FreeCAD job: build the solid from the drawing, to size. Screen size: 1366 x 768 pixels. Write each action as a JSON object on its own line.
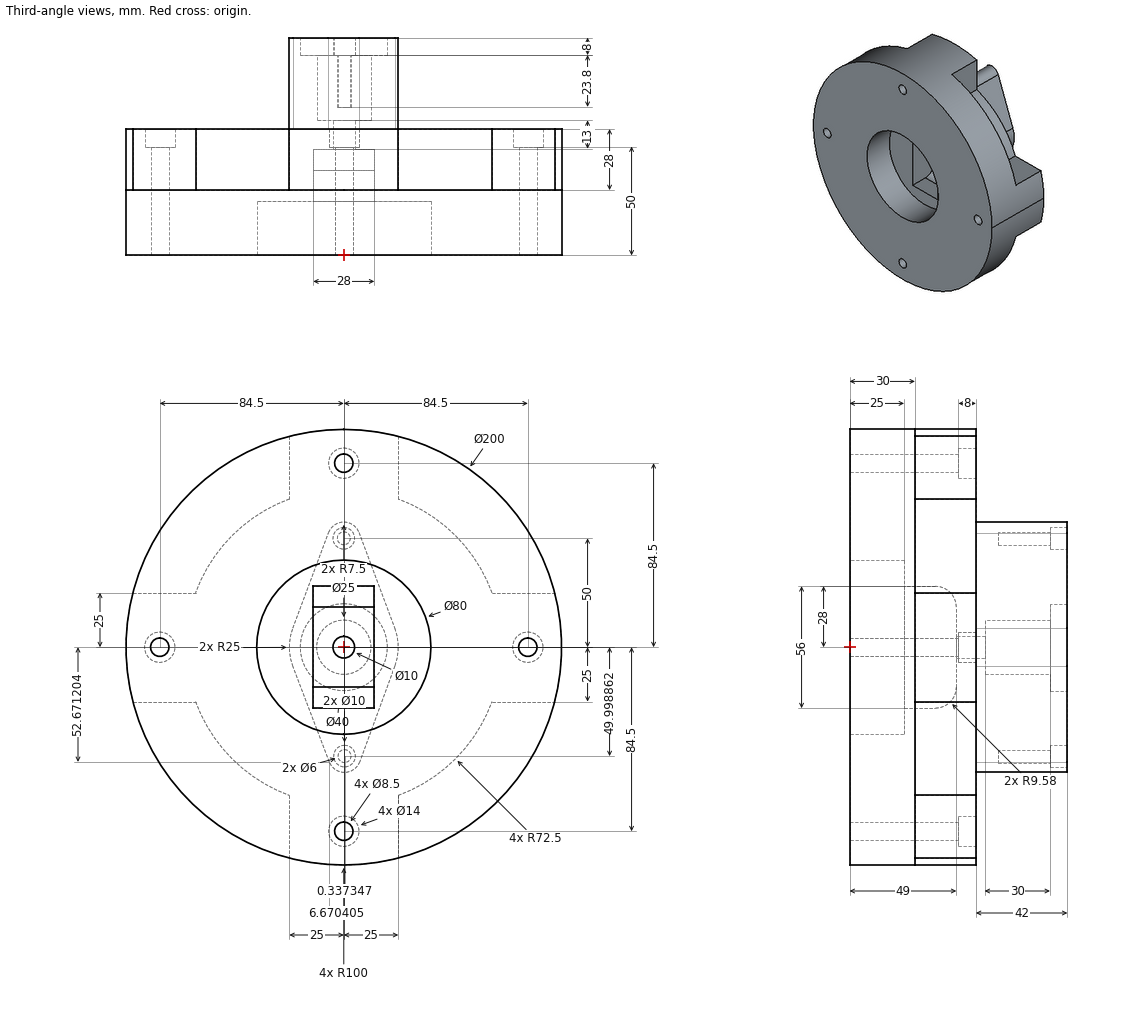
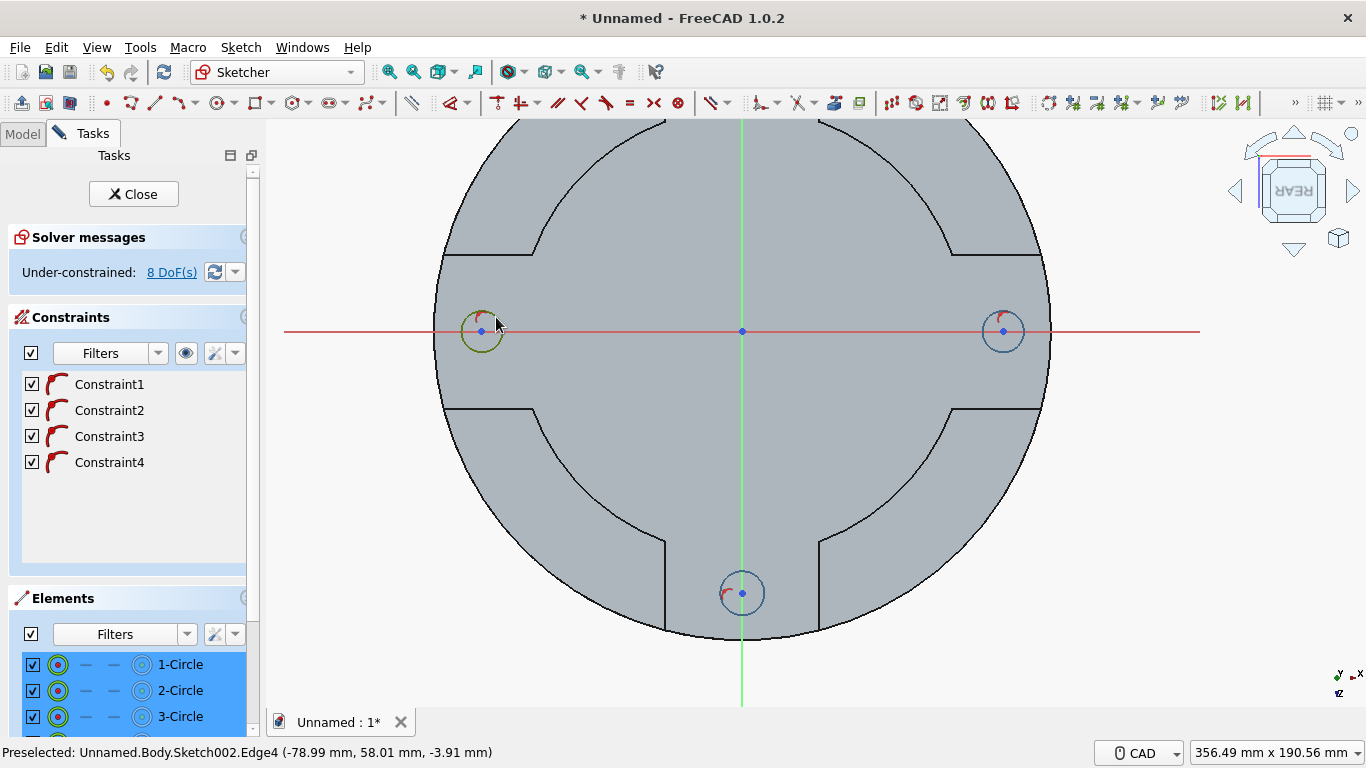
{"action": "key", "text": "e"}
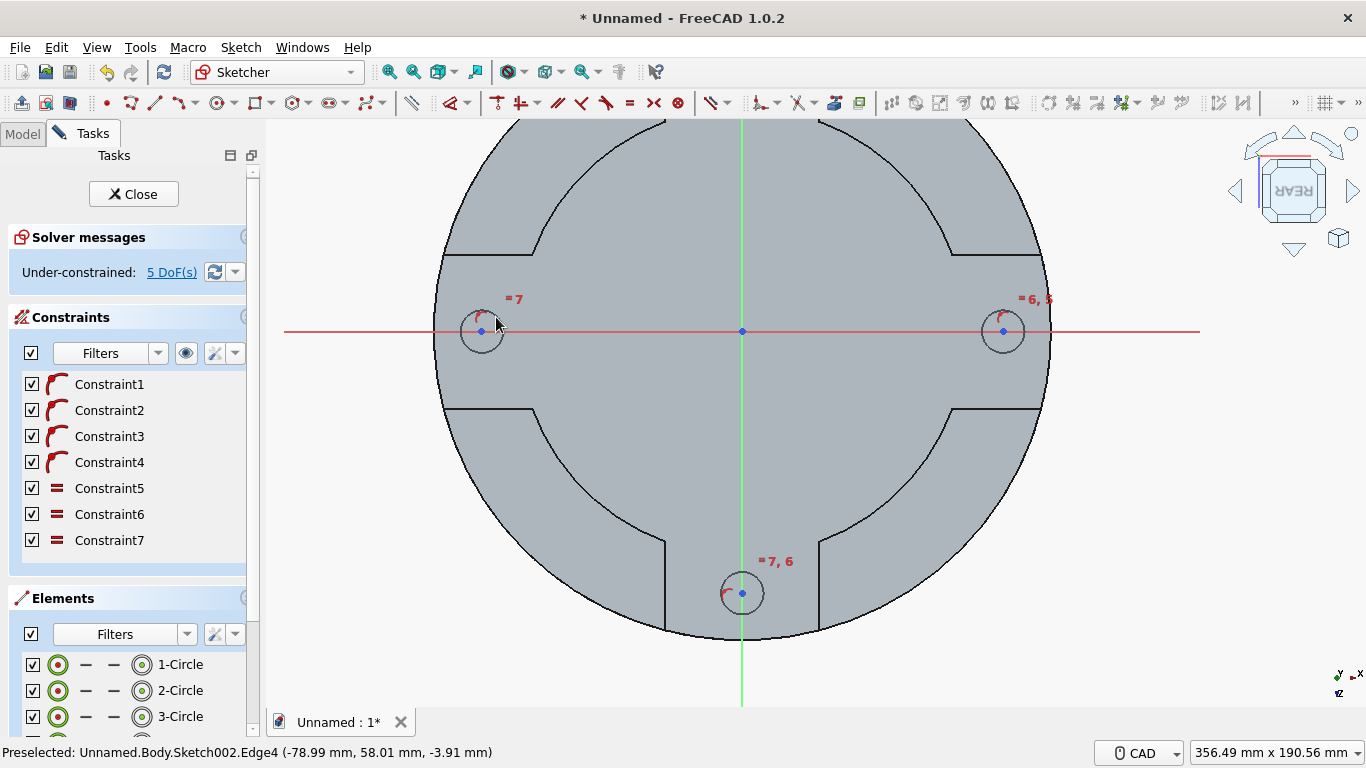
{"action": "left_click", "coordinate": [450, 104]}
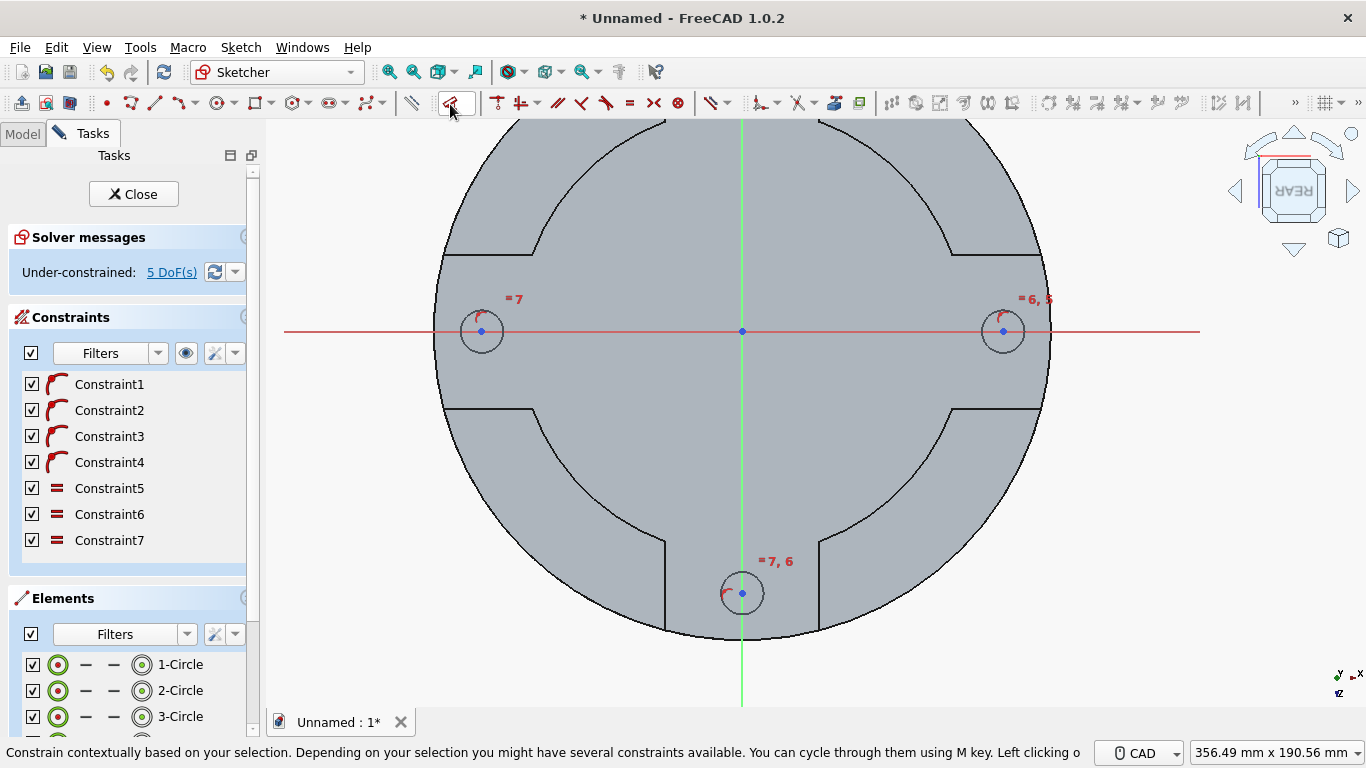
{"action": "scroll", "coordinate": [758, 578], "scroll_direction": "down", "scroll_amount": 2}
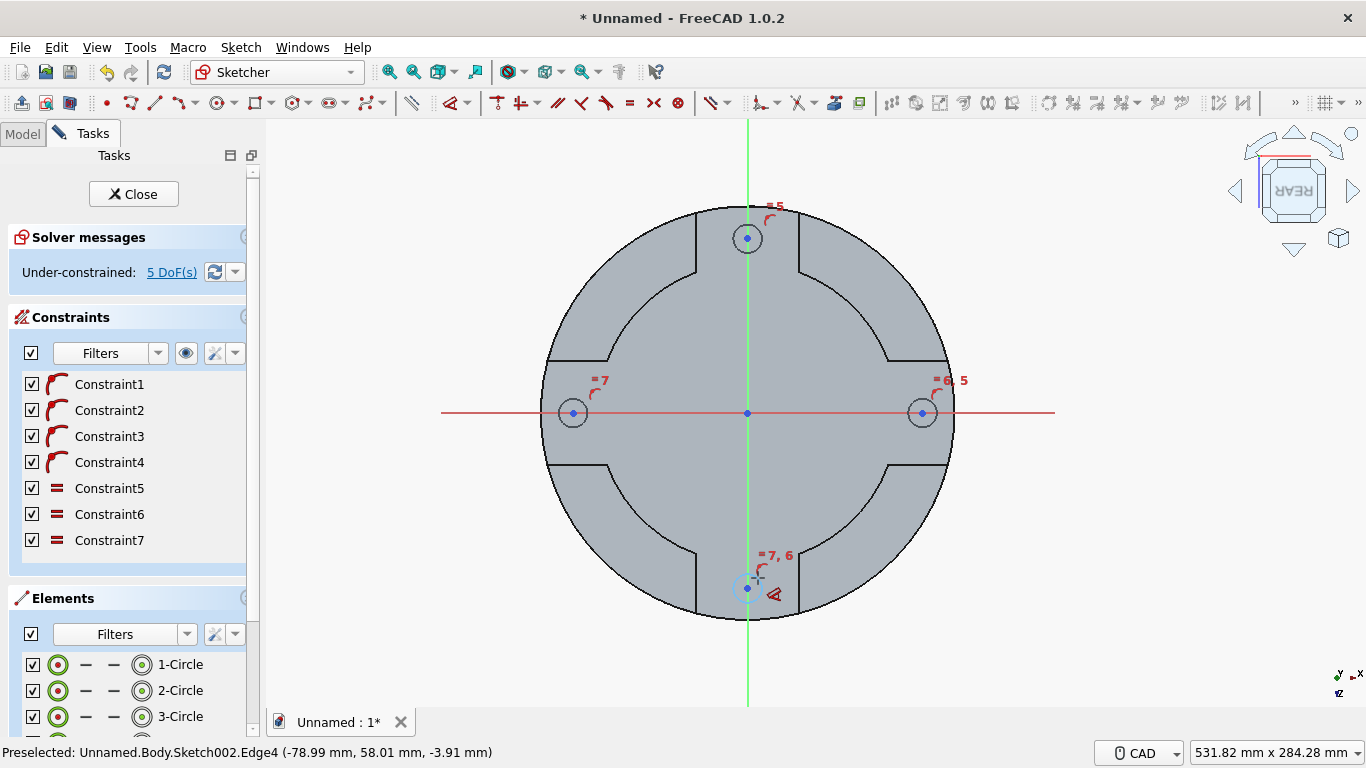
{"action": "scroll", "coordinate": [758, 229], "scroll_direction": "up", "scroll_amount": 2}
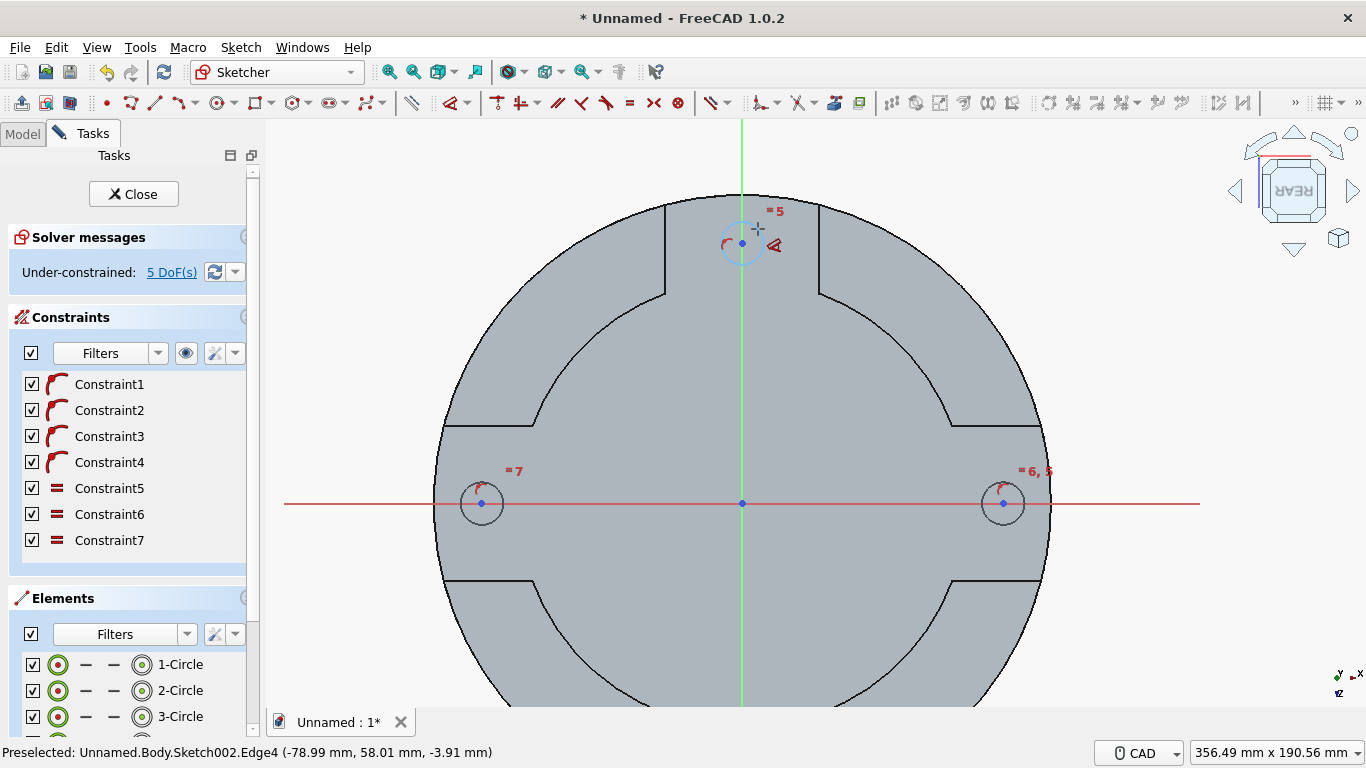
{"action": "left_click", "coordinate": [757, 228]}
{"action": "left_click", "coordinate": [779, 205]}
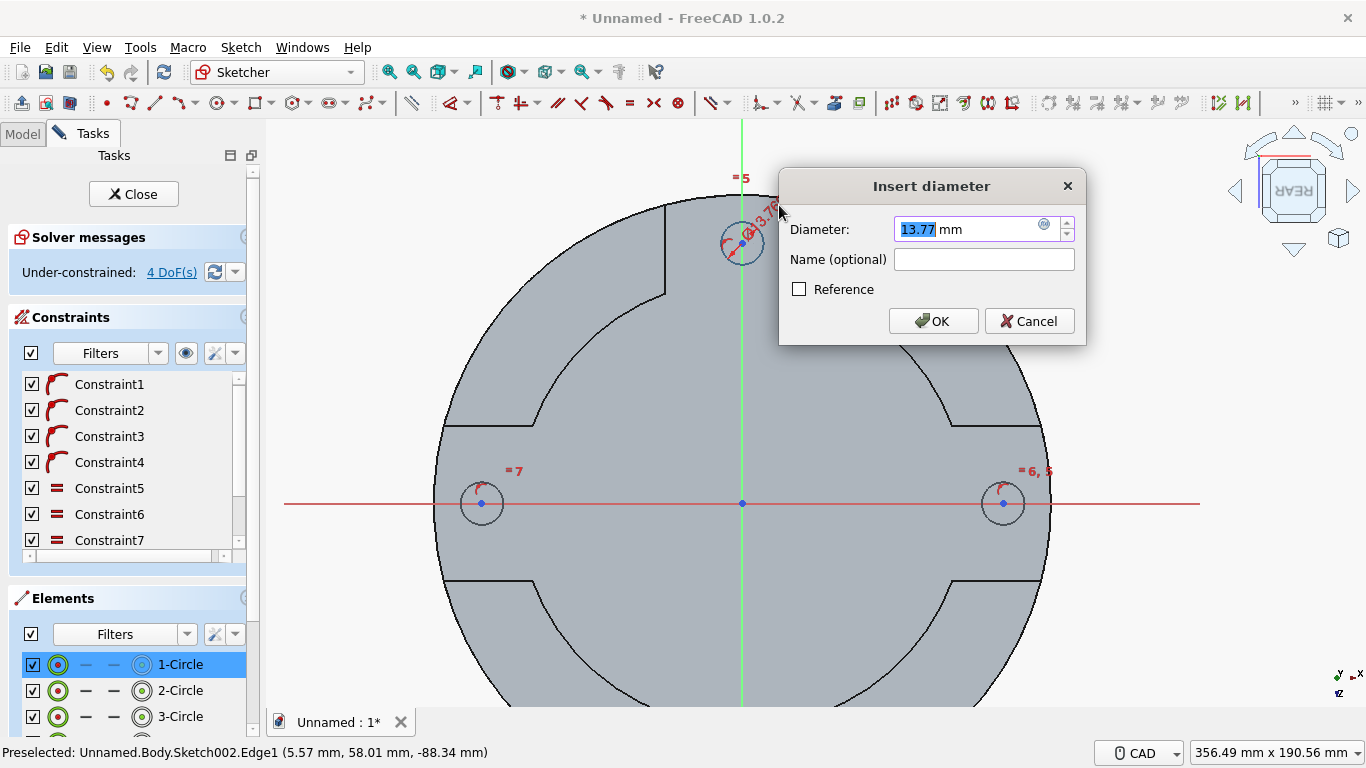
{"action": "type", "text": "14"}
{"action": "key", "text": "Return"}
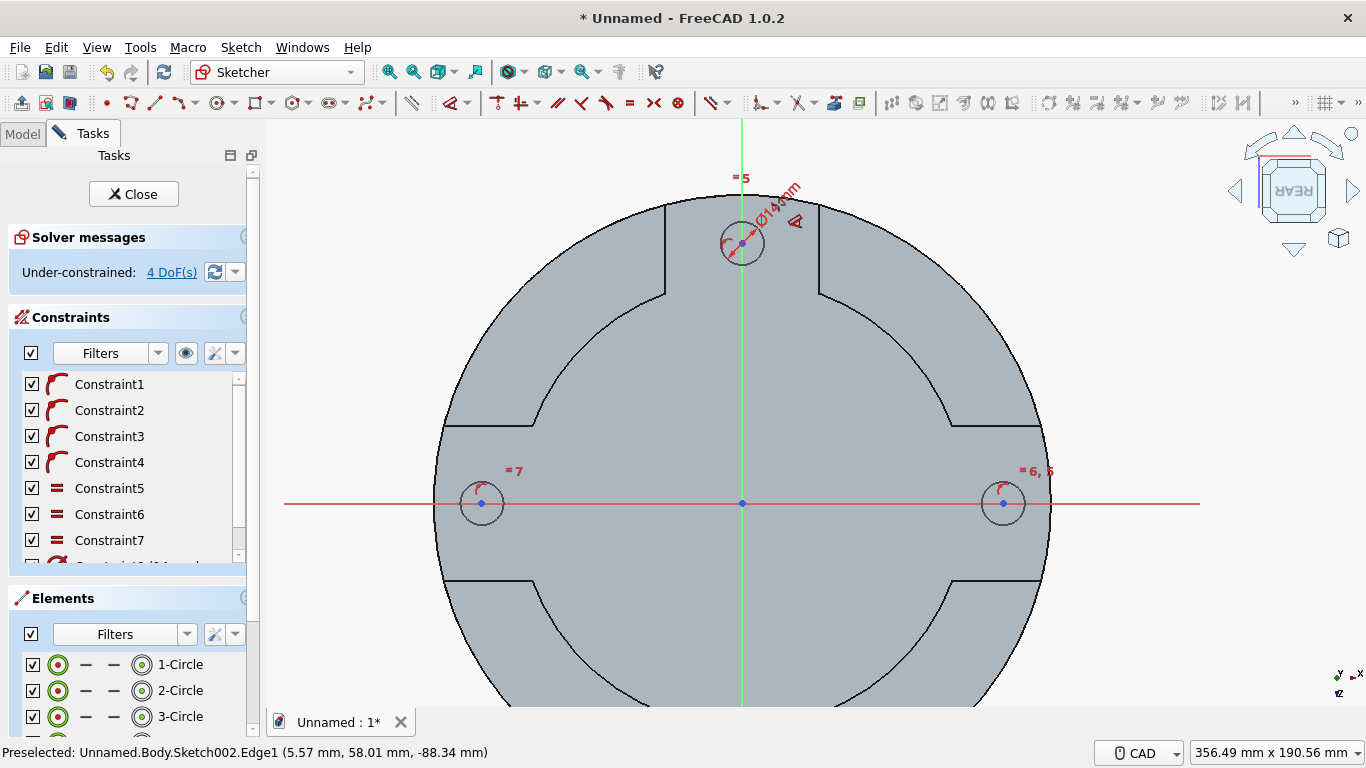
{"action": "left_click", "coordinate": [742, 243]}
{"action": "left_click", "coordinate": [776, 374]}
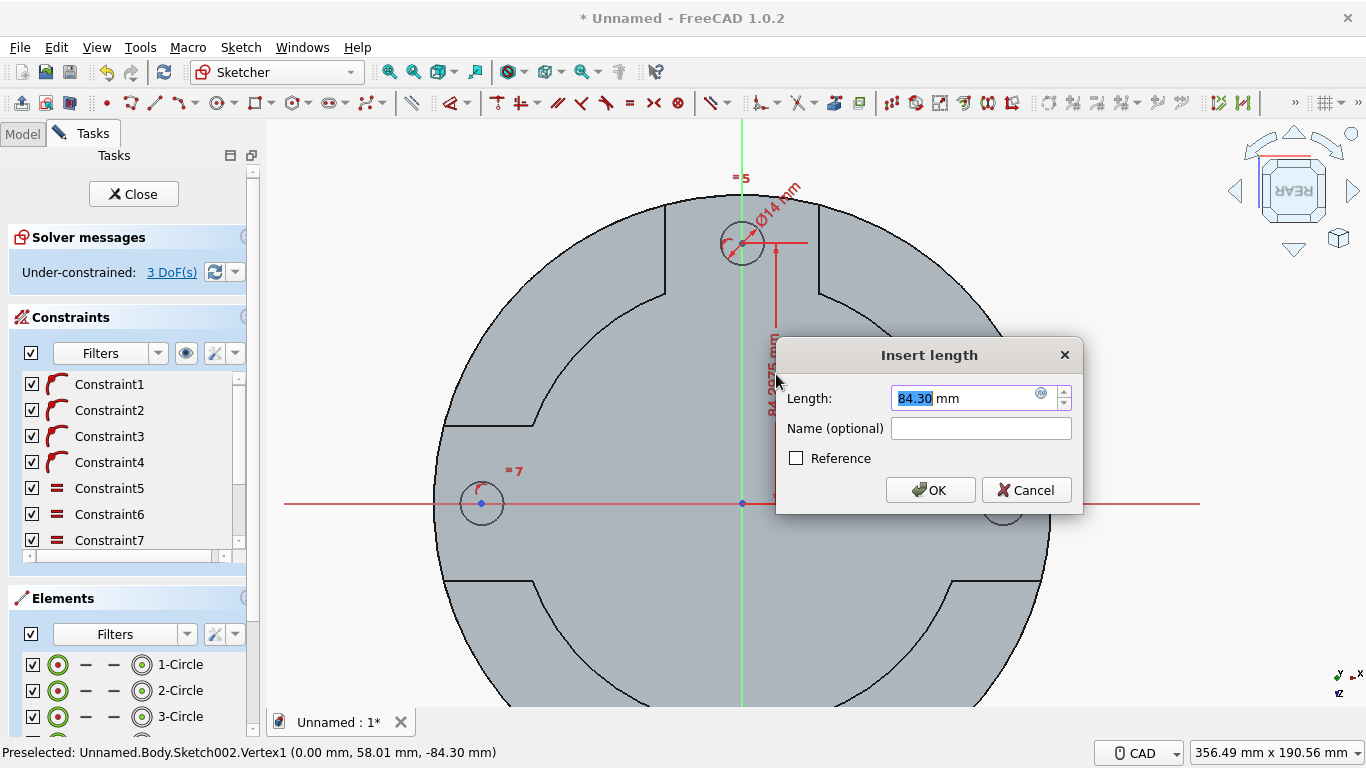
{"action": "type", "text": "84.5"}
{"action": "key", "text": "Return"}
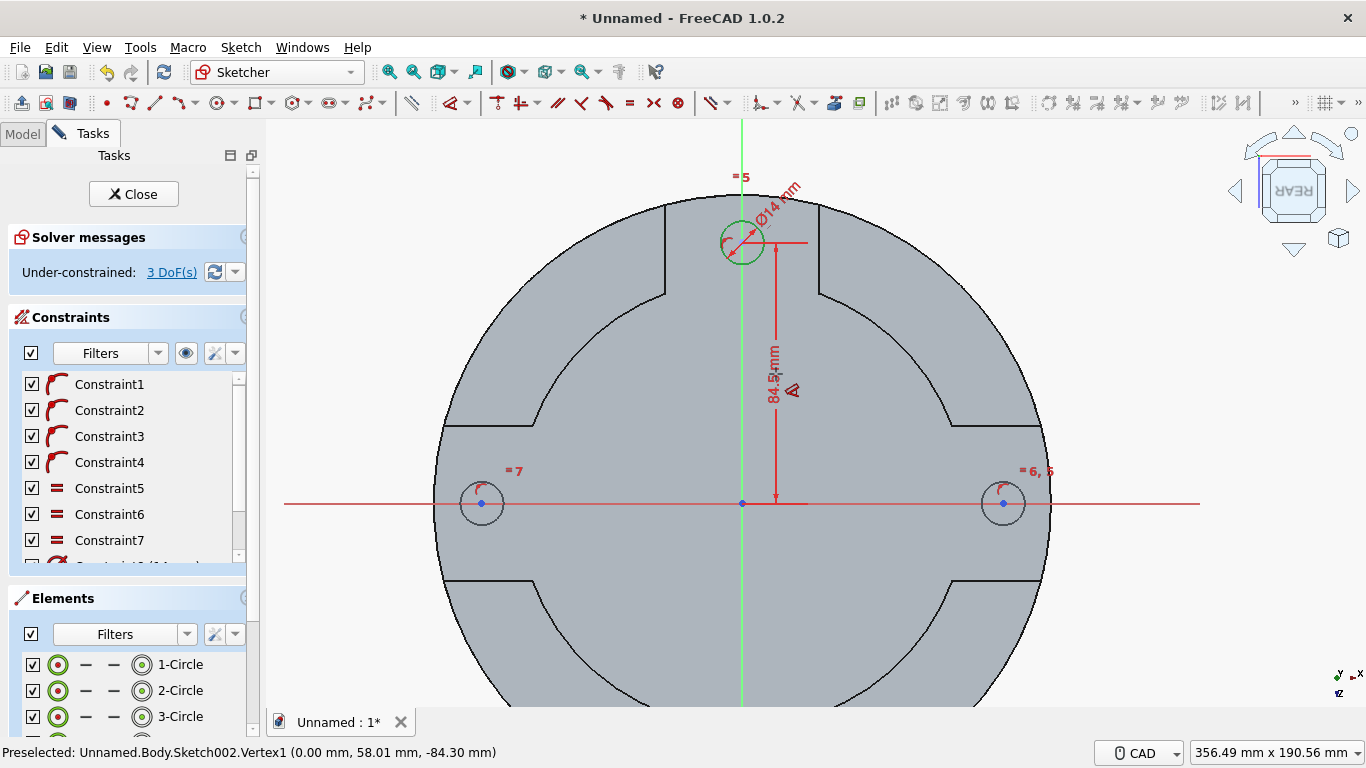
{"action": "left_click", "coordinate": [1003, 504]}
{"action": "left_click", "coordinate": [873, 538]}